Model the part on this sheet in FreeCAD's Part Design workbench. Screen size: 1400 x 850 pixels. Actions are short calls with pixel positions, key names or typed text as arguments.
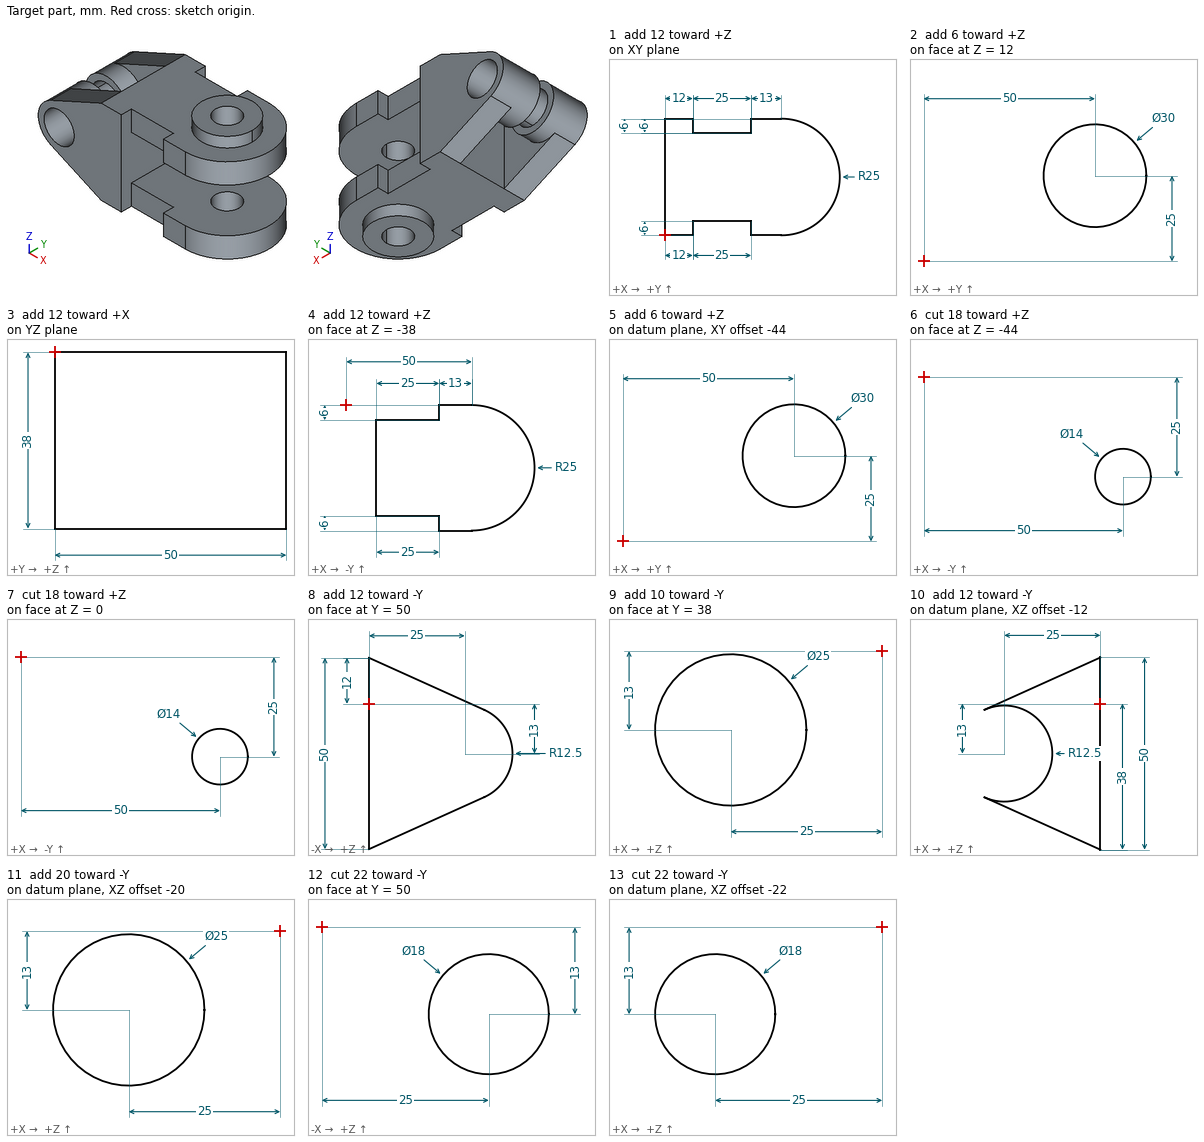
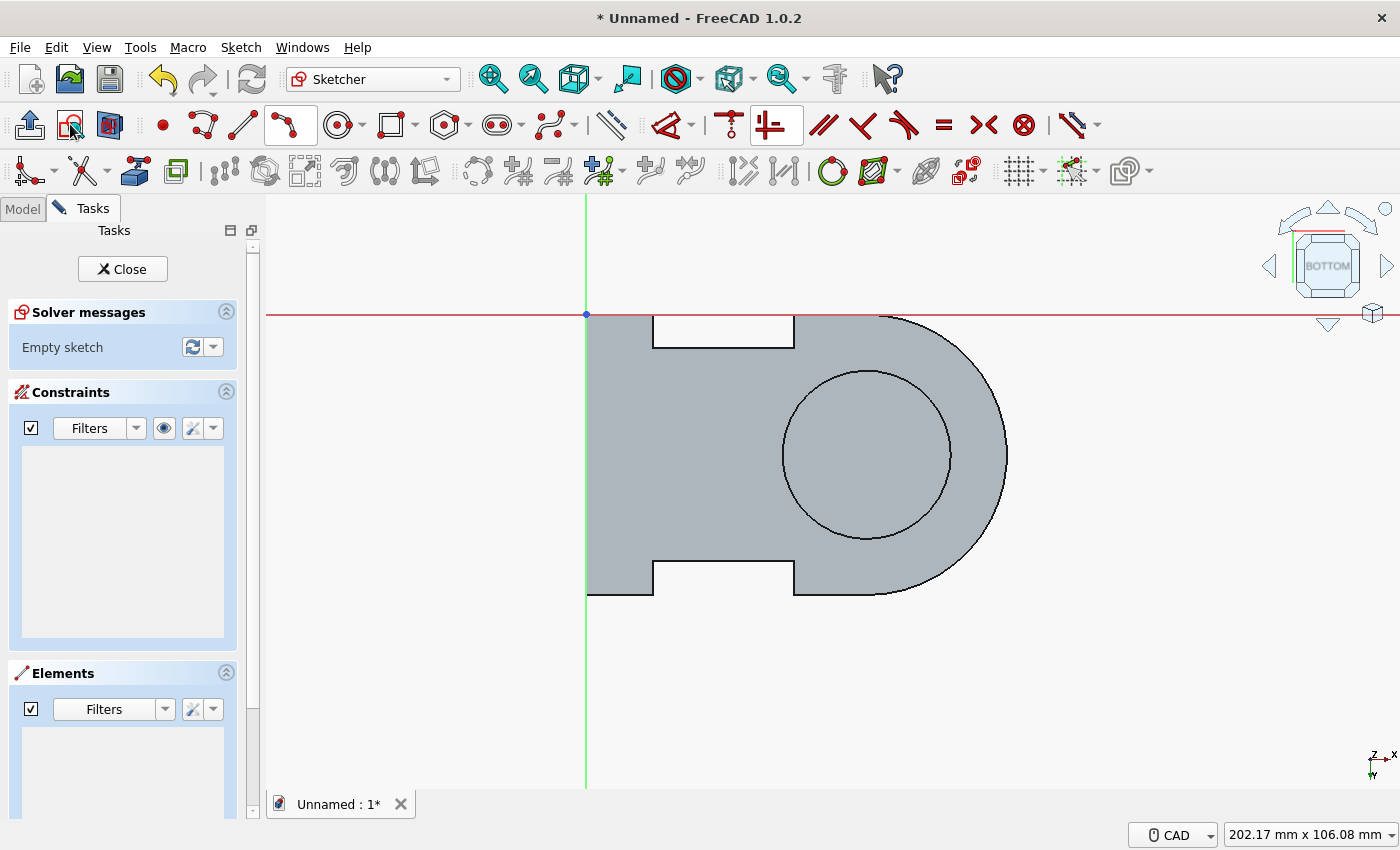
scroll(892, 446, up, 8)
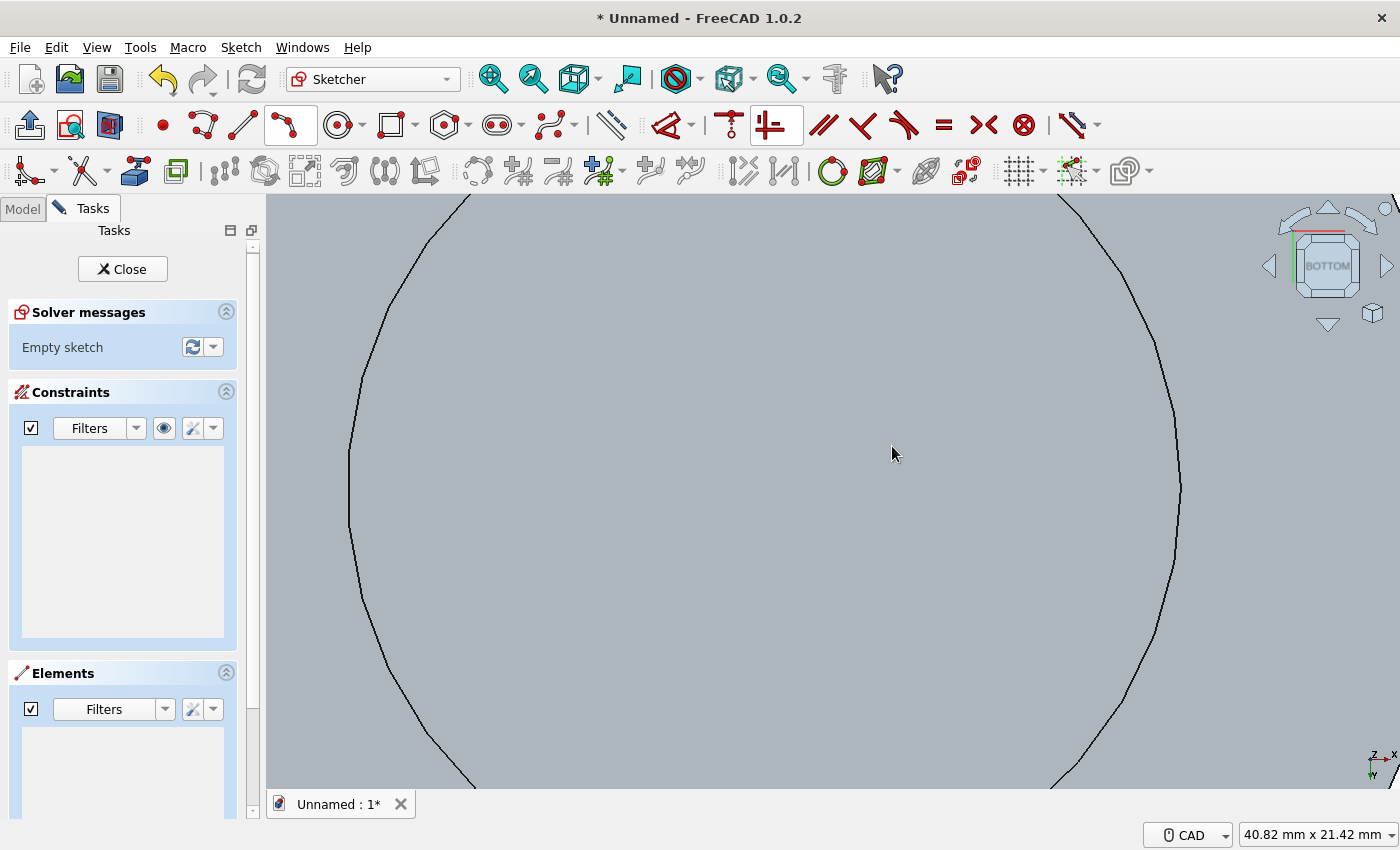
click(338, 126)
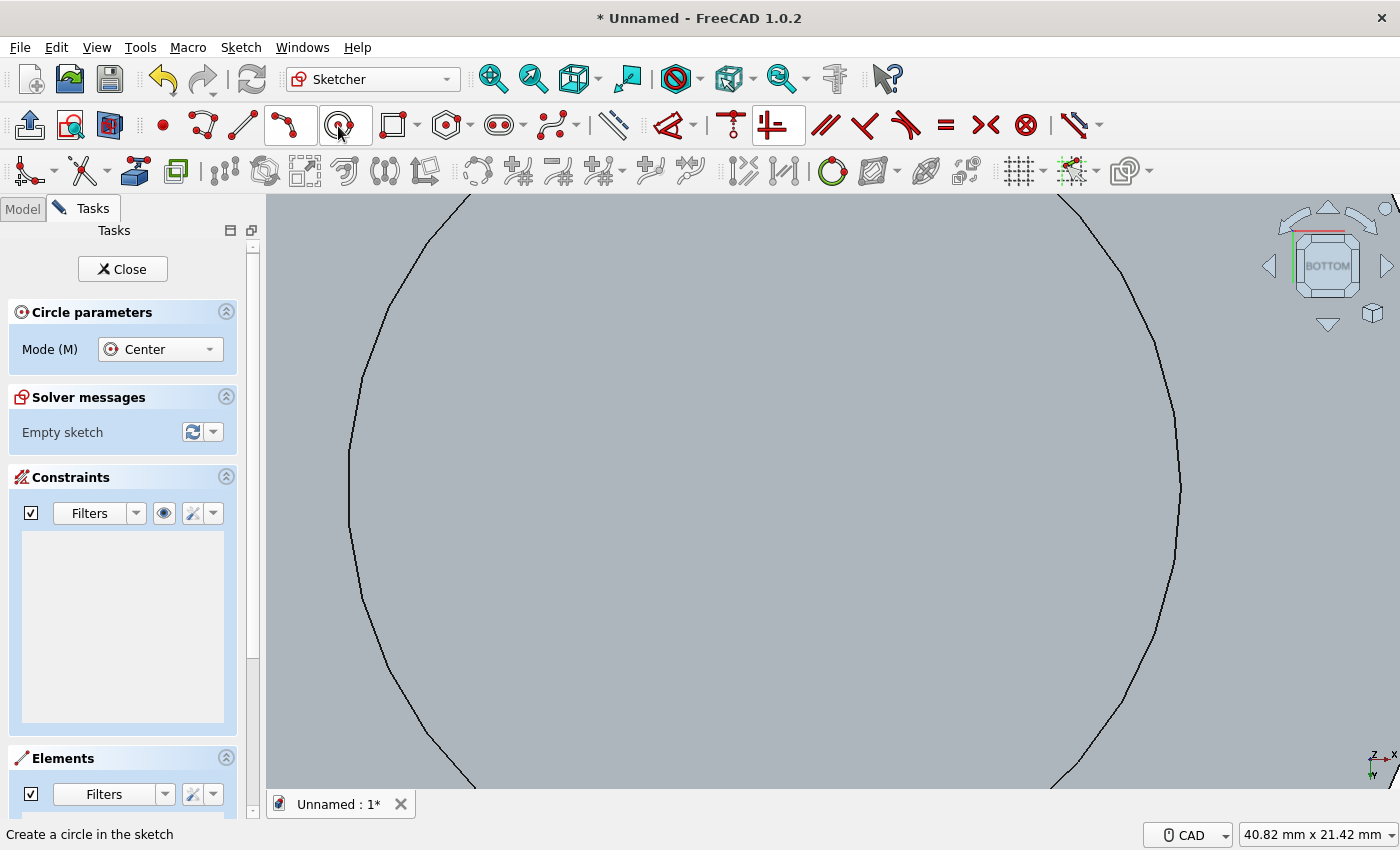
click(764, 488)
click(902, 351)
key(Escape)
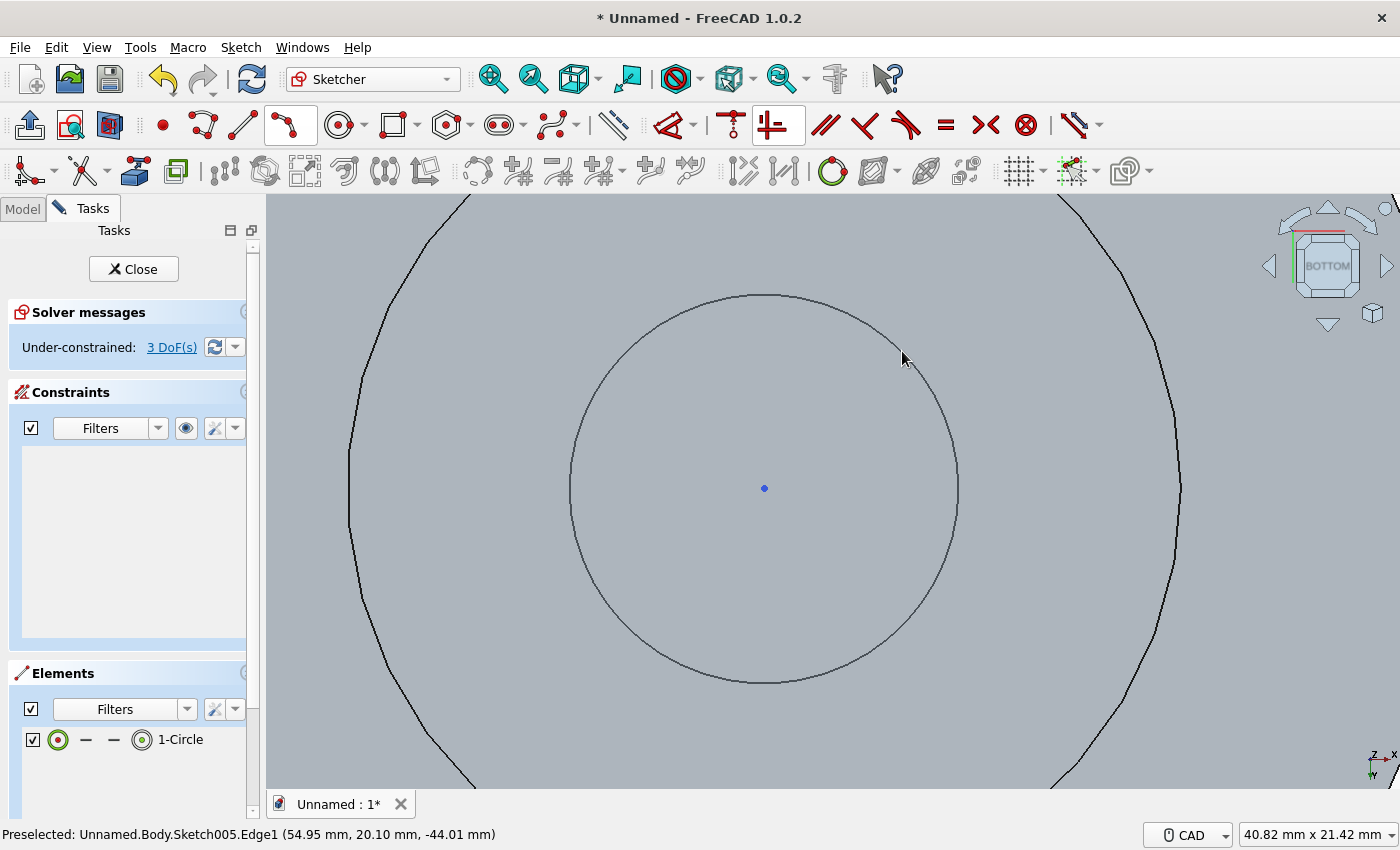
key(d)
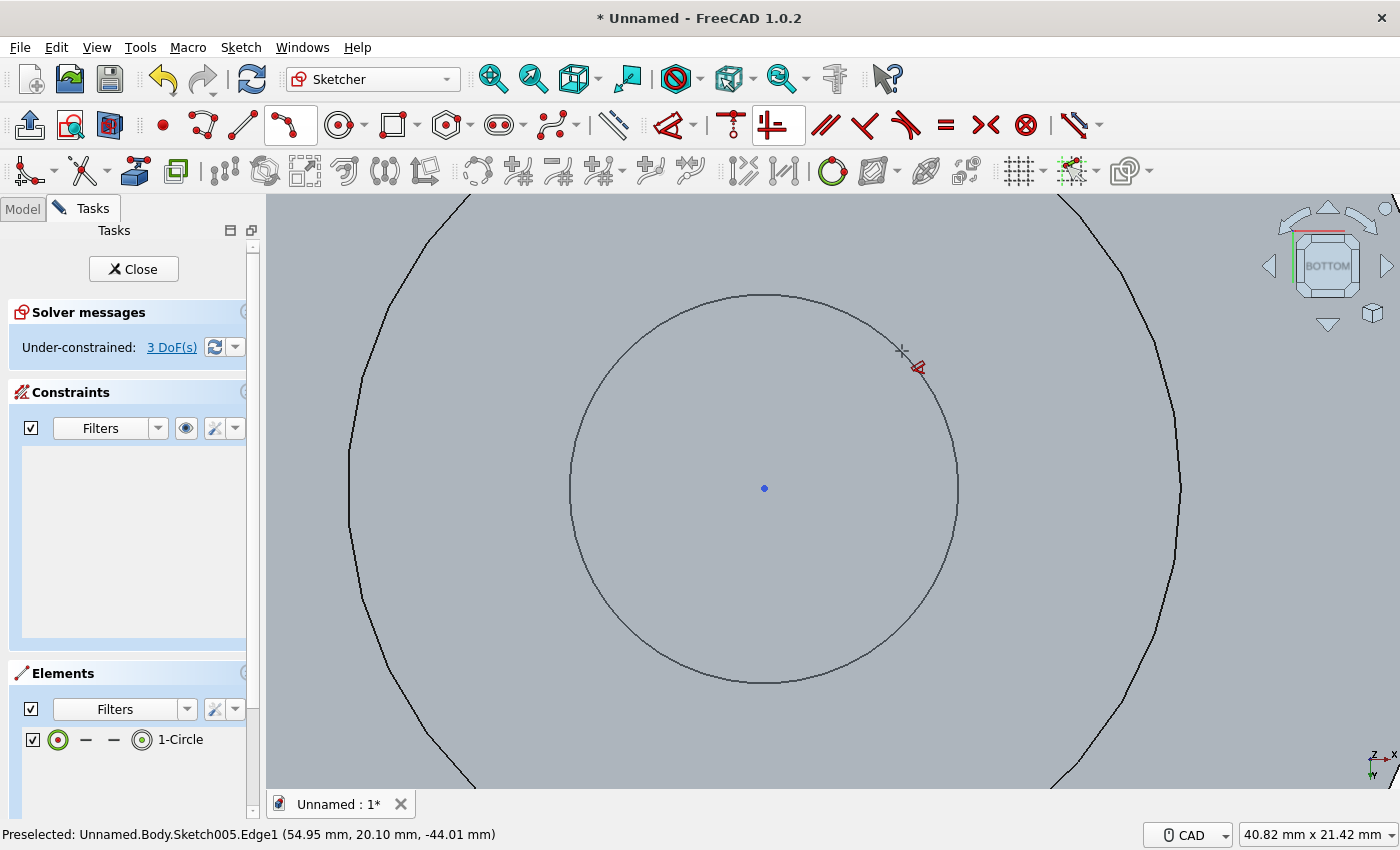
click(901, 351)
click(924, 328)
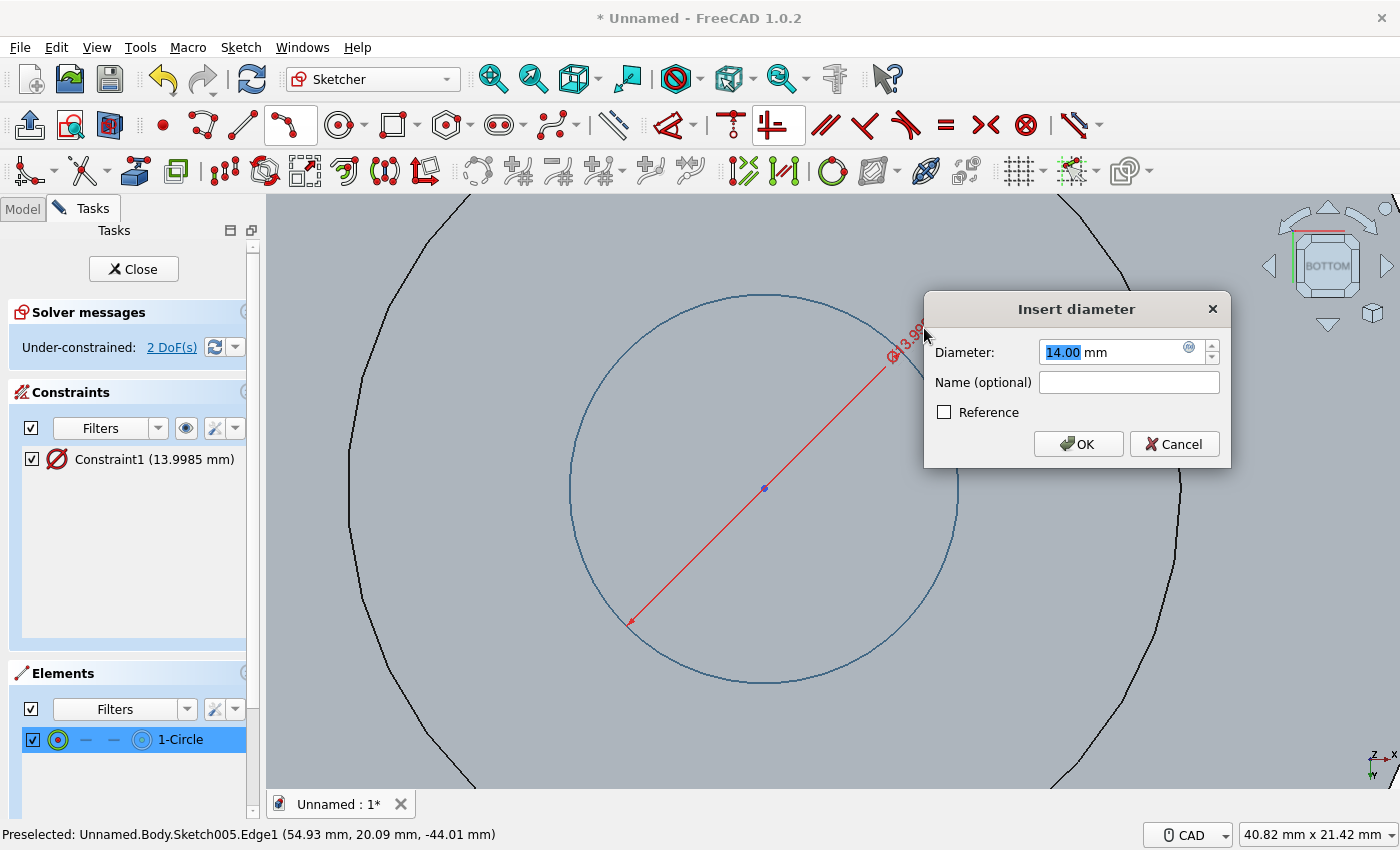
text(14)
key(Return)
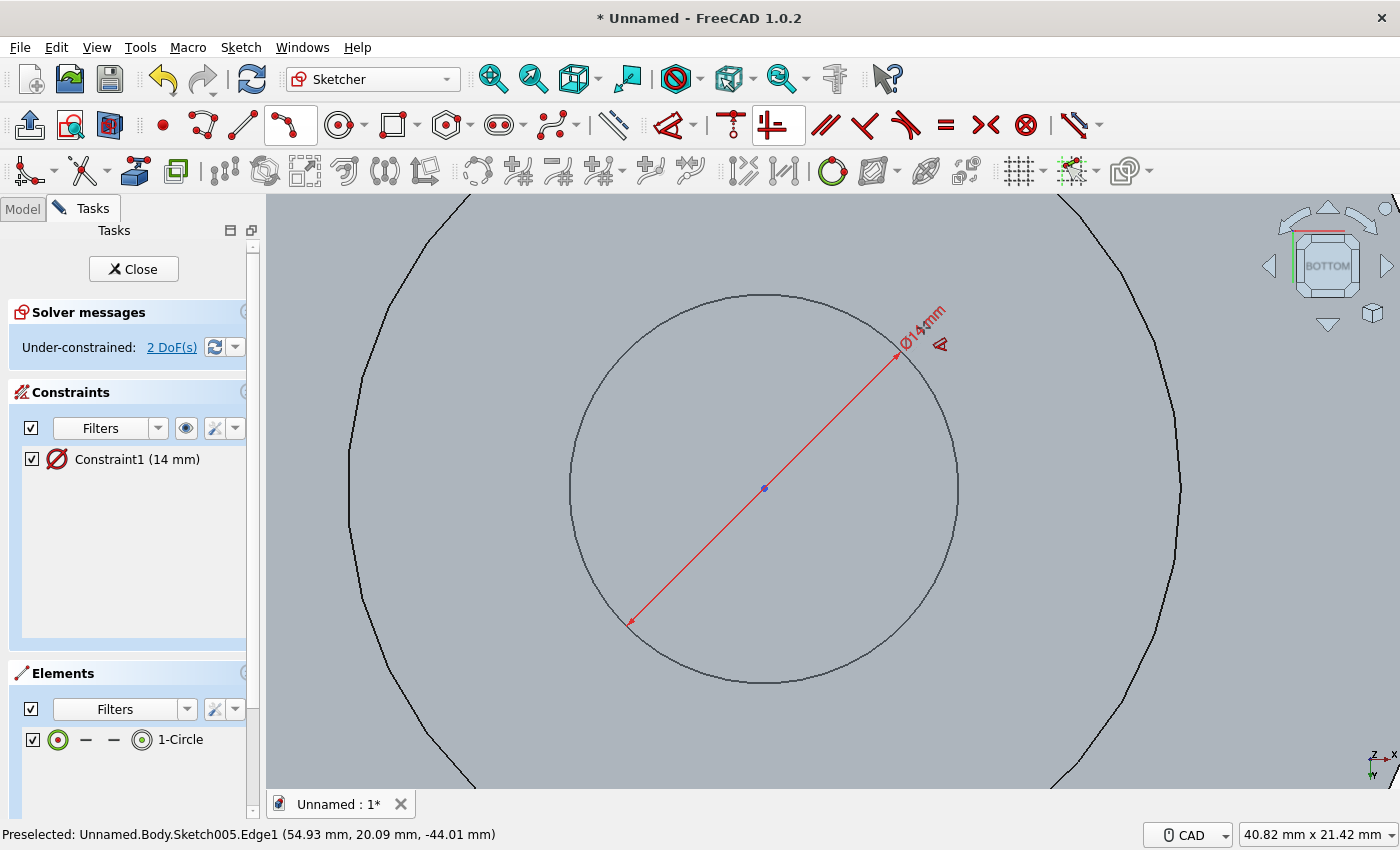
click(764, 489)
click(529, 523)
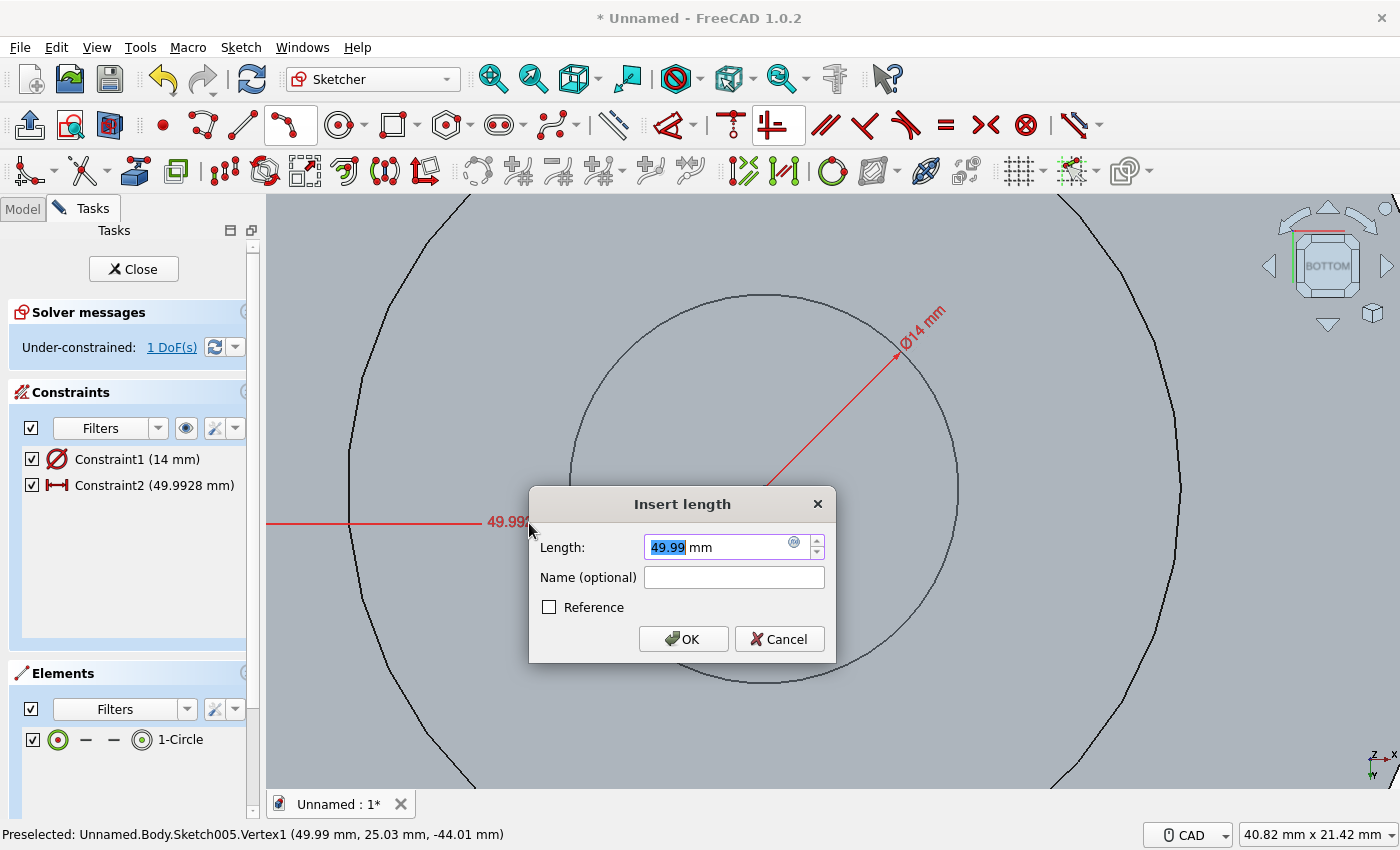
text(50)
key(Return)